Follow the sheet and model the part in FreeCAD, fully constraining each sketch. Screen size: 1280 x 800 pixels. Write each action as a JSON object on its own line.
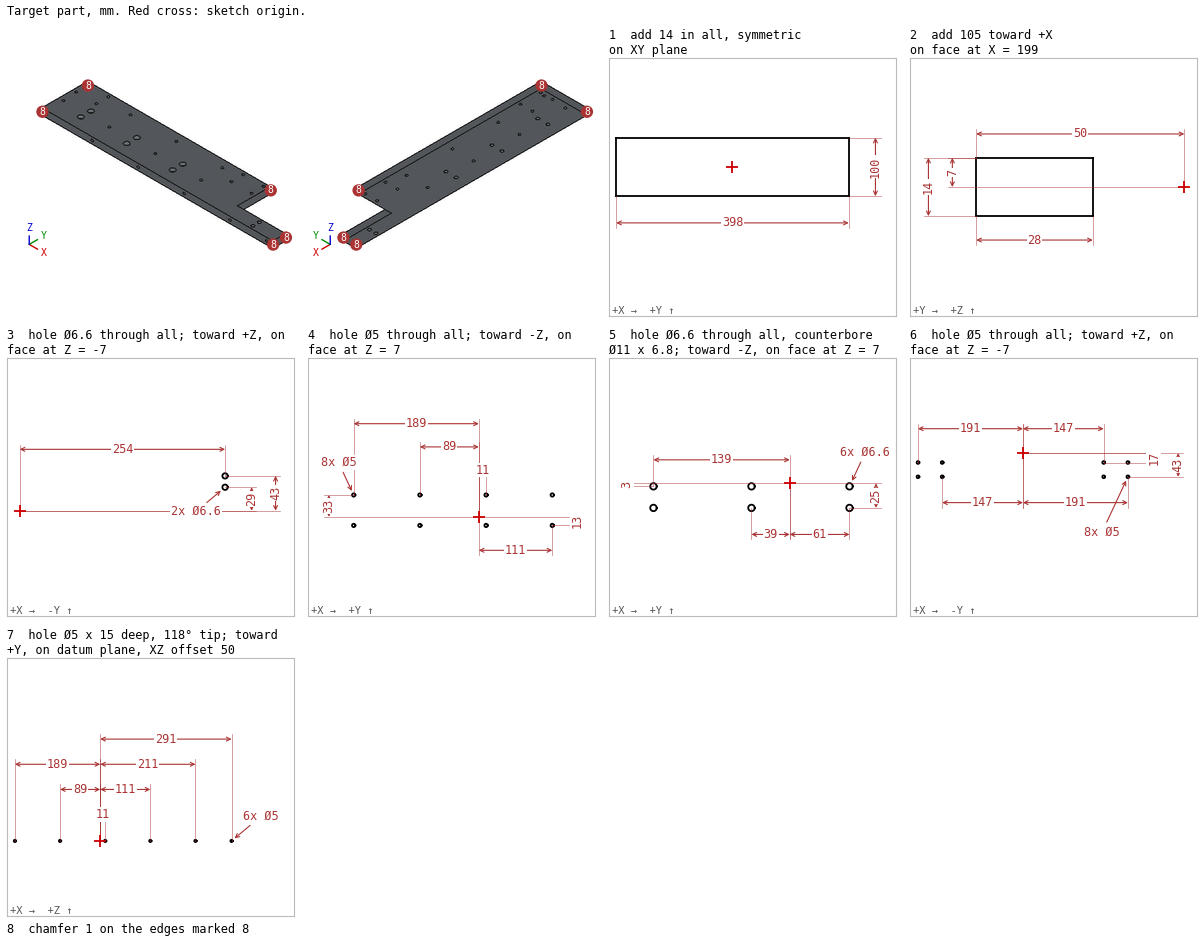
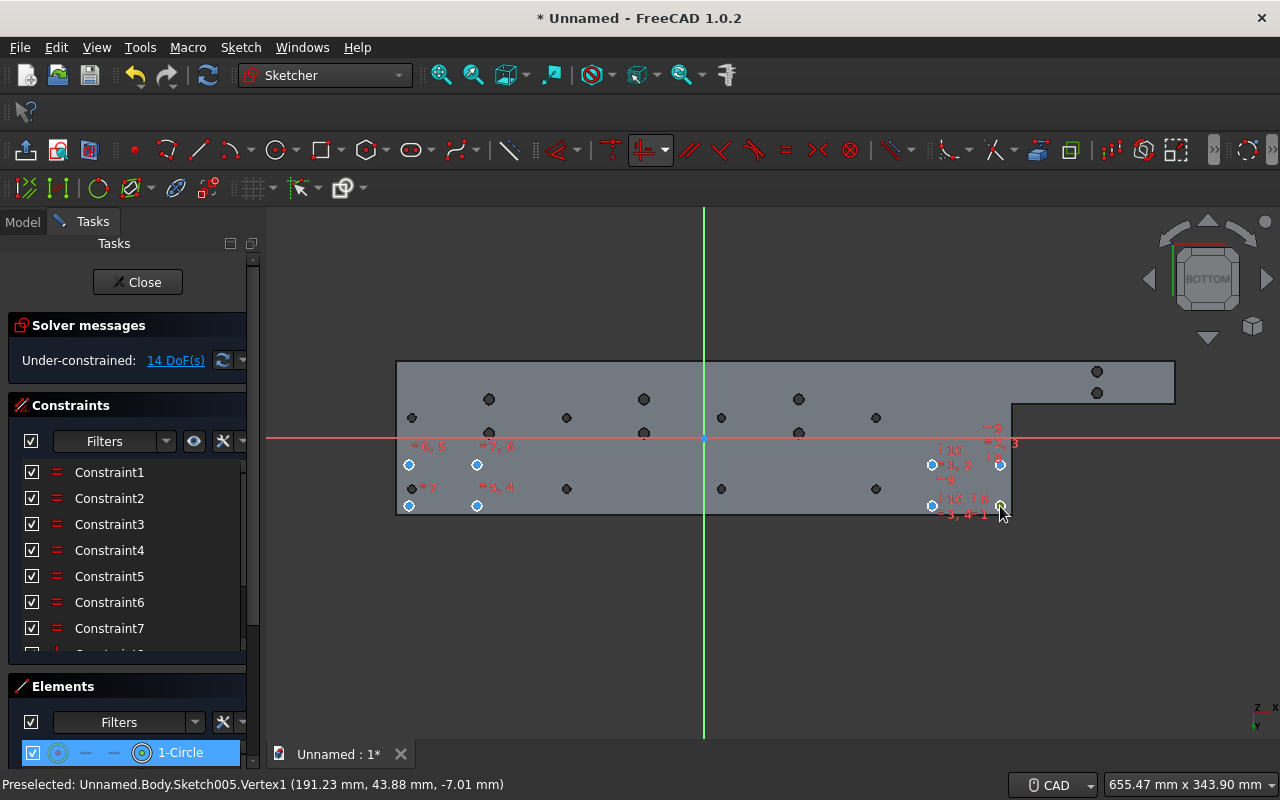
{"action": "left_click", "coordinate": [932, 506]}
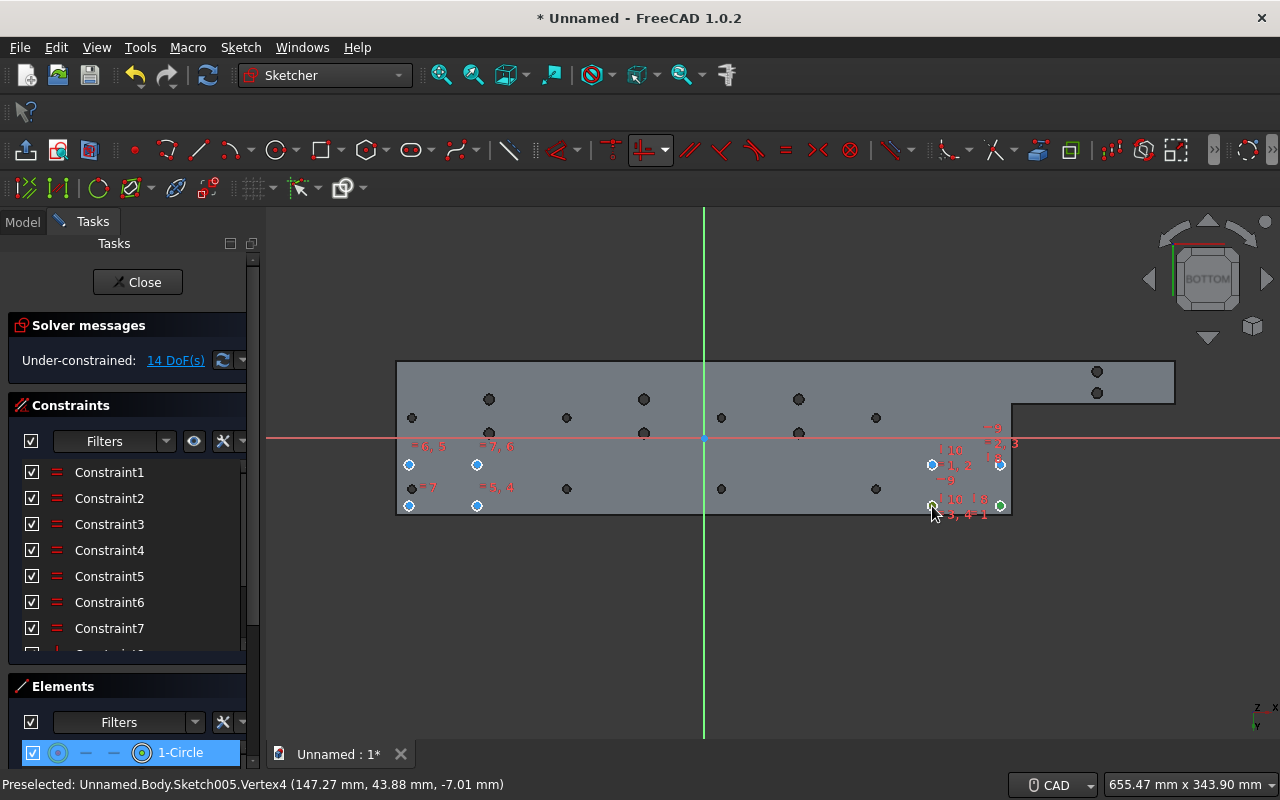
{"action": "key", "text": "h"}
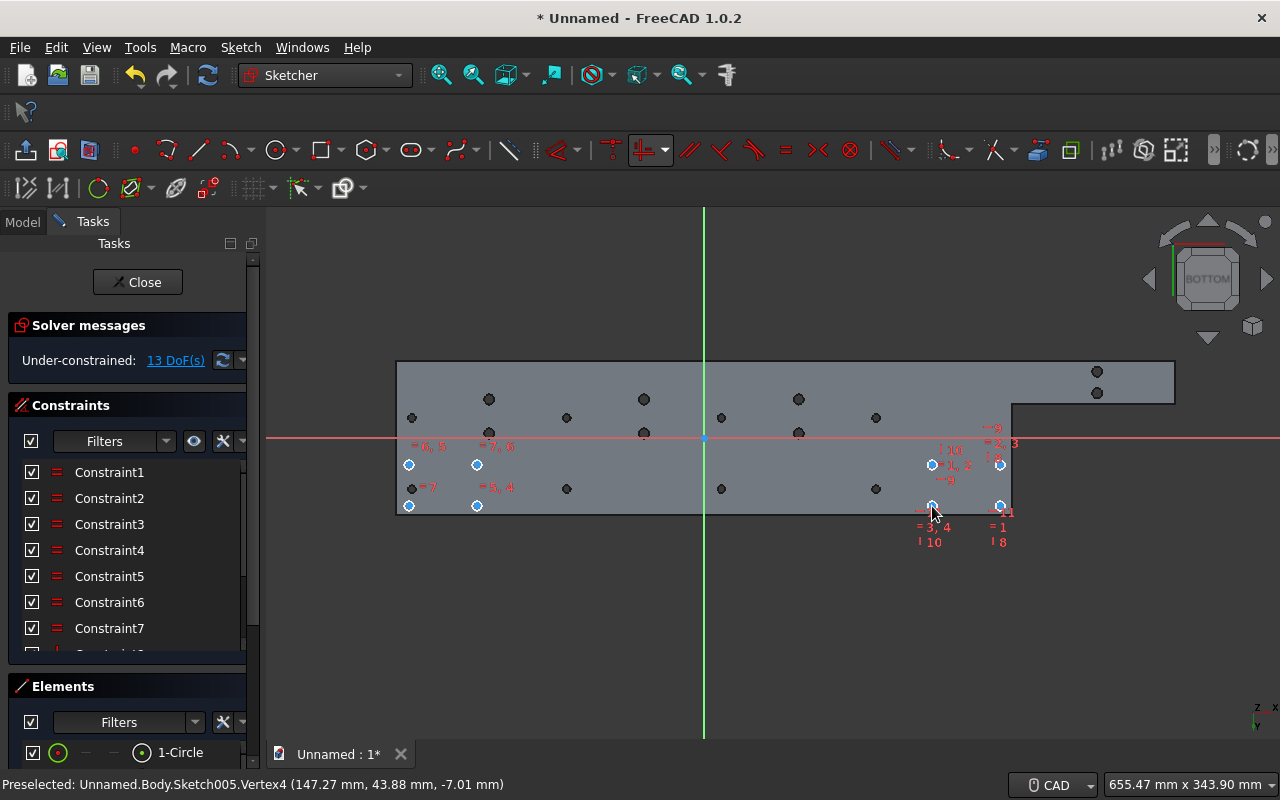
{"action": "scroll", "coordinate": [932, 506], "scroll_direction": "up", "scroll_amount": 4}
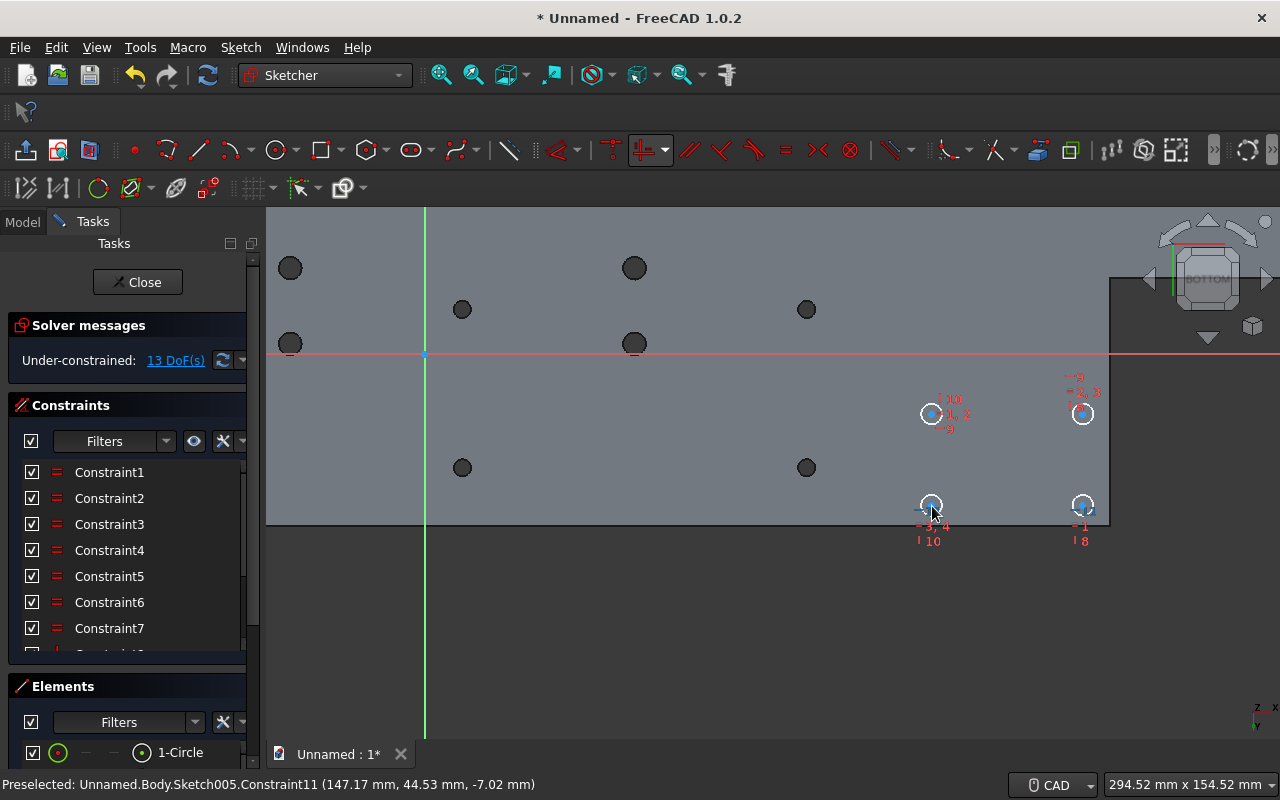
{"action": "left_click", "coordinate": [930, 503]}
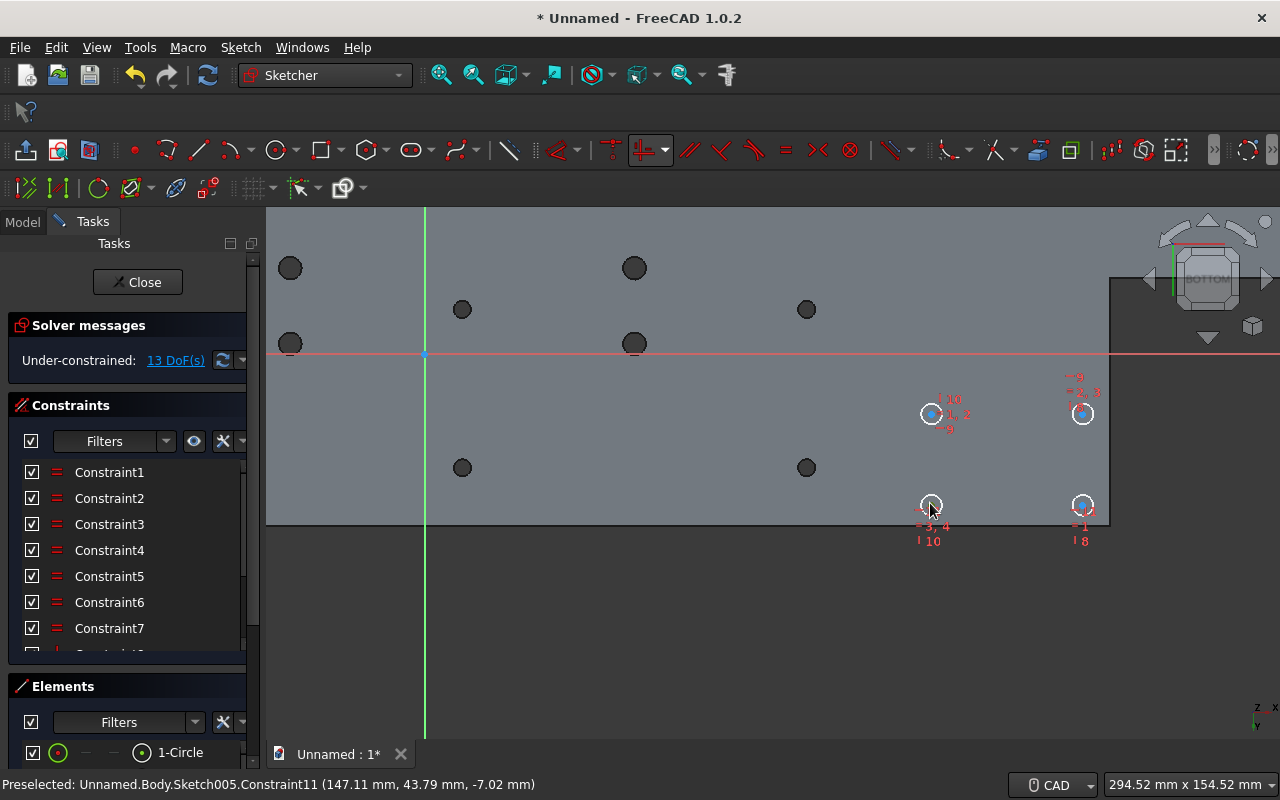
{"action": "scroll", "coordinate": [933, 506], "scroll_direction": "down", "scroll_amount": 4}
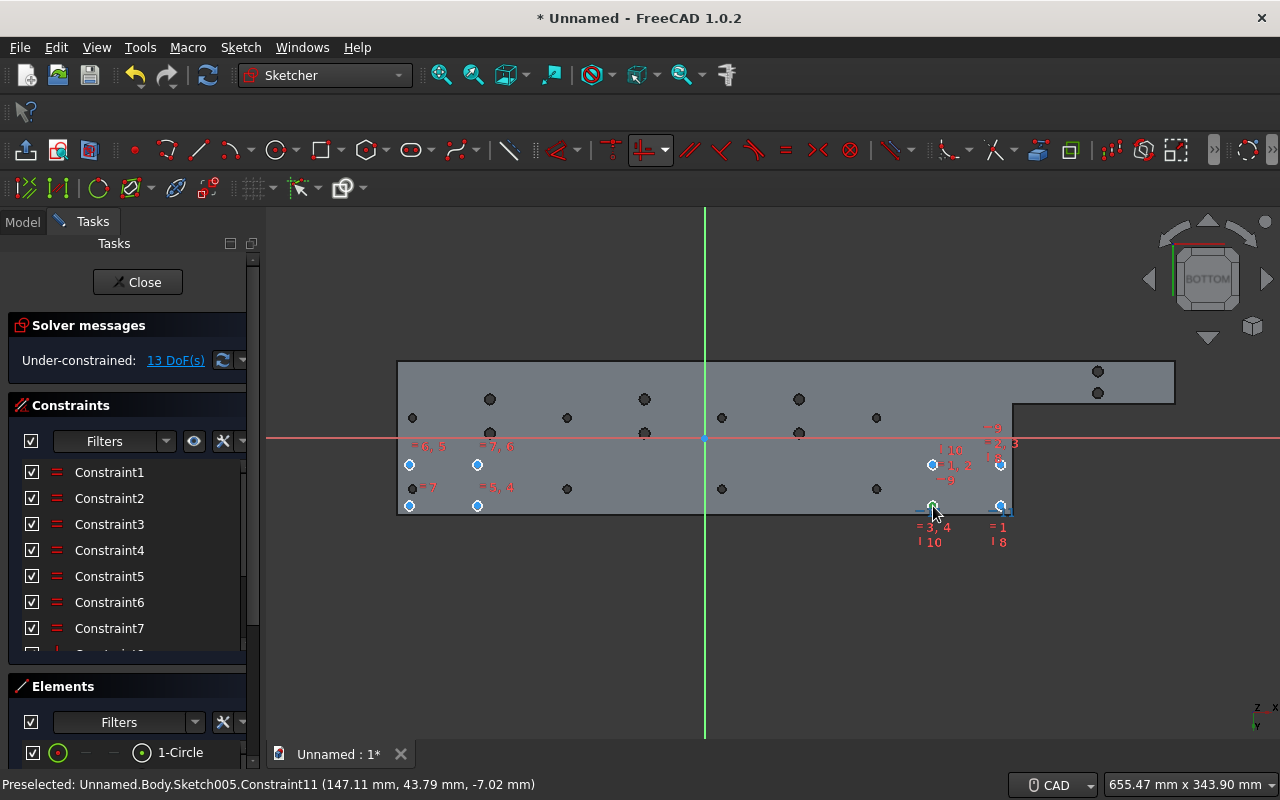
{"action": "left_click", "coordinate": [478, 506]}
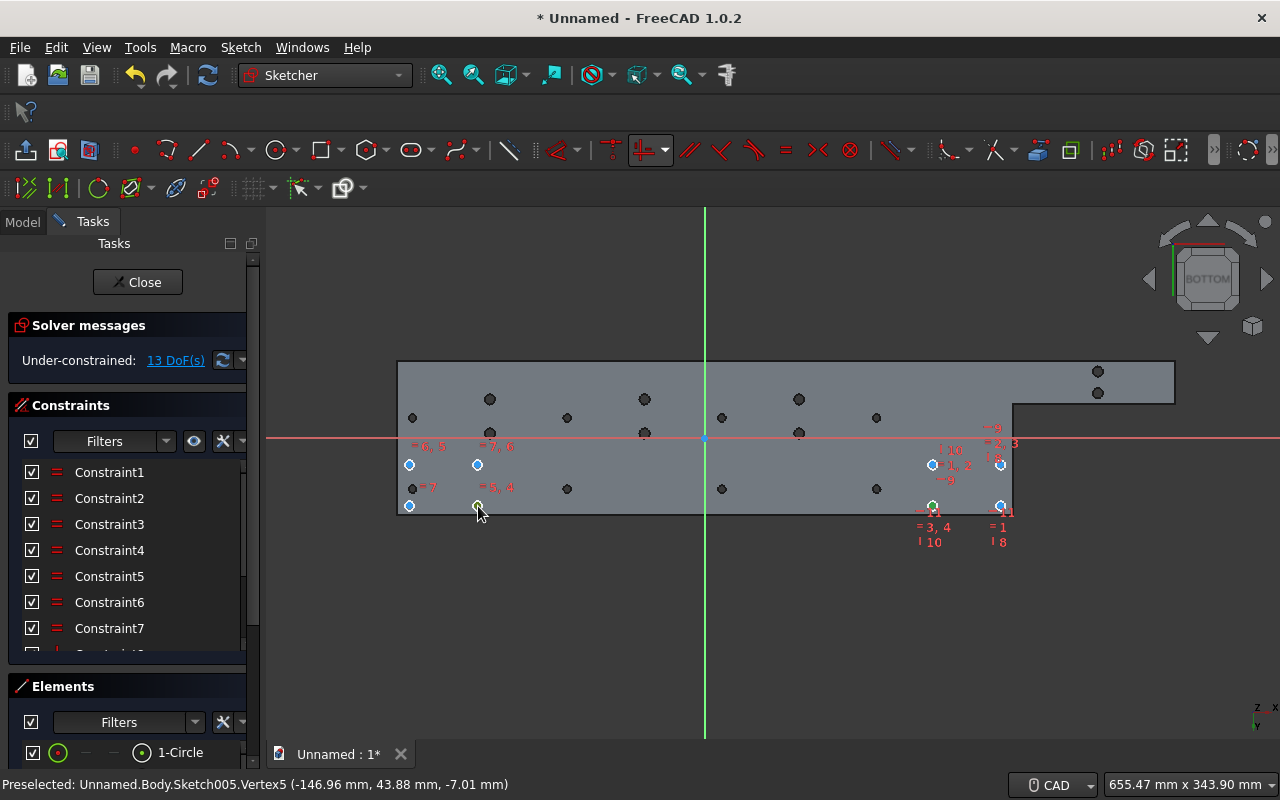
{"action": "left_click", "coordinate": [668, 150]}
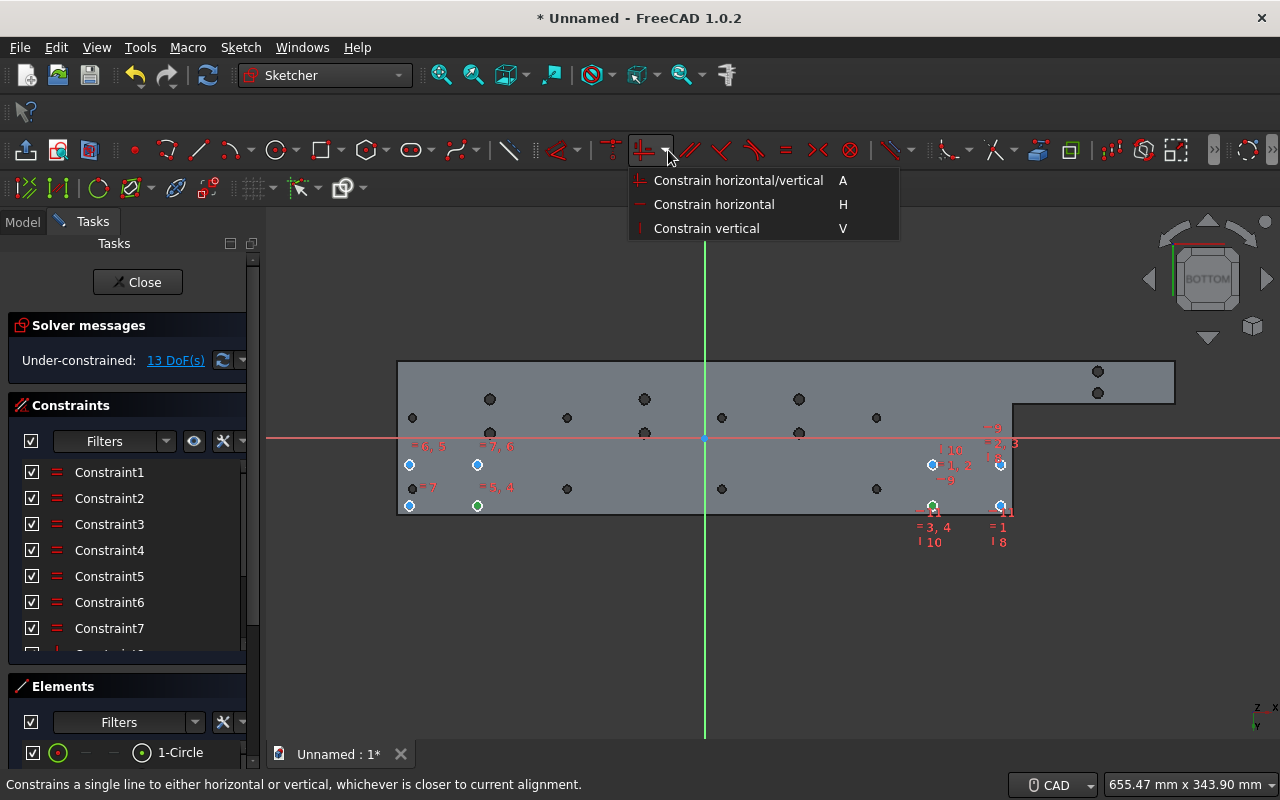
{"action": "left_click", "coordinate": [764, 204]}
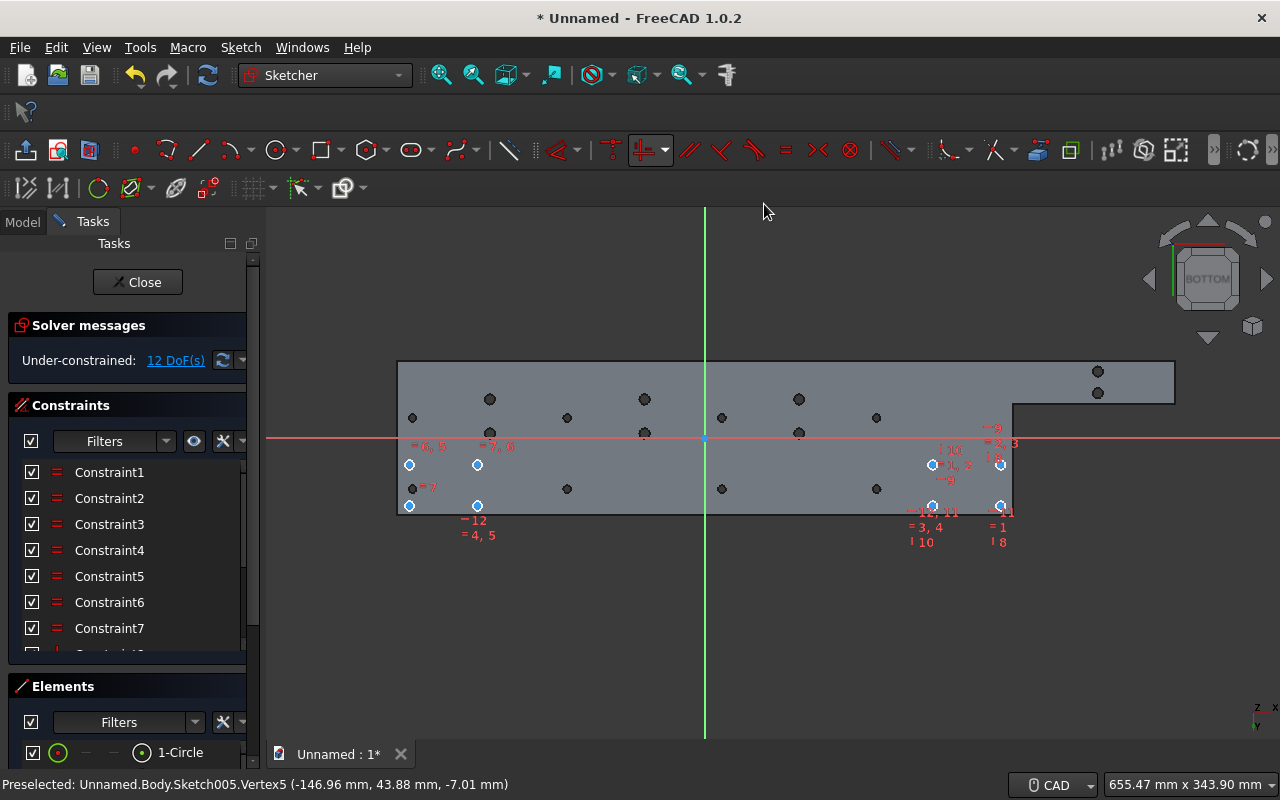
{"action": "left_click", "coordinate": [933, 465]}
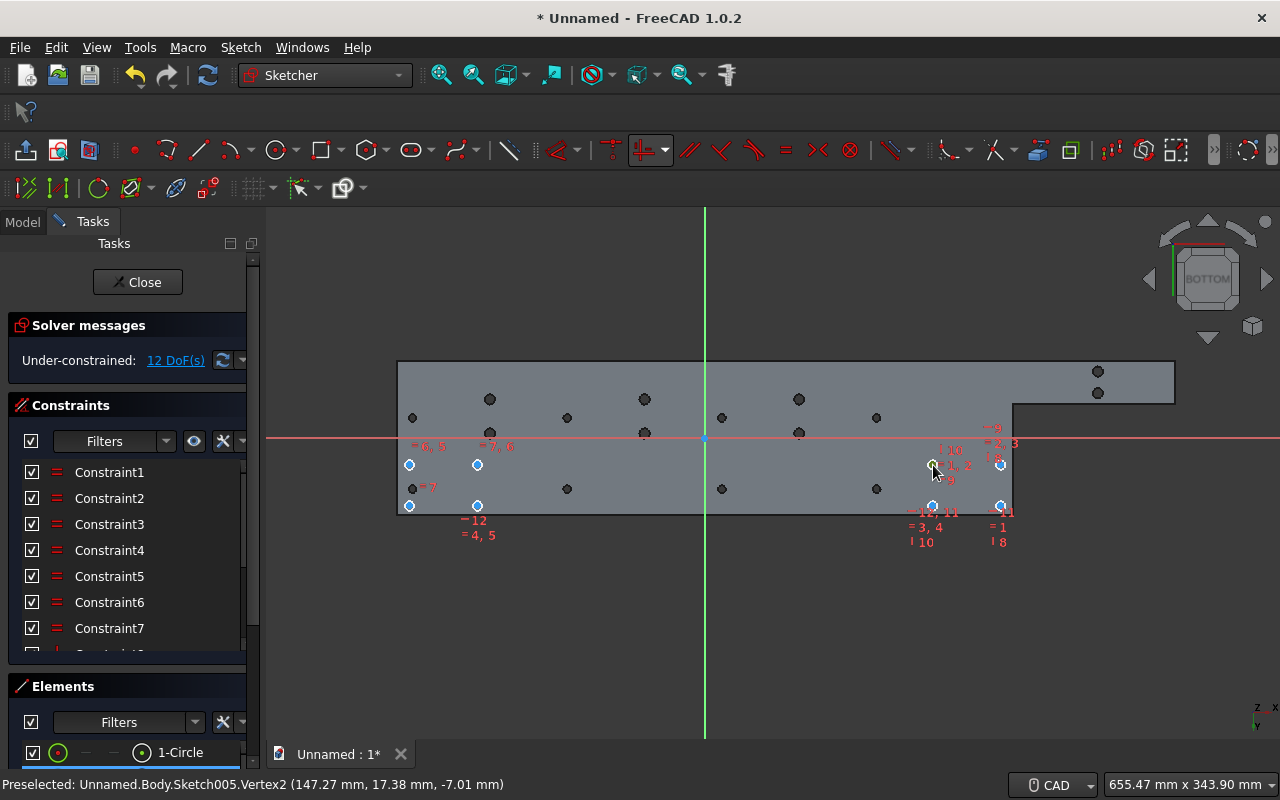
{"action": "left_click", "coordinate": [410, 465]}